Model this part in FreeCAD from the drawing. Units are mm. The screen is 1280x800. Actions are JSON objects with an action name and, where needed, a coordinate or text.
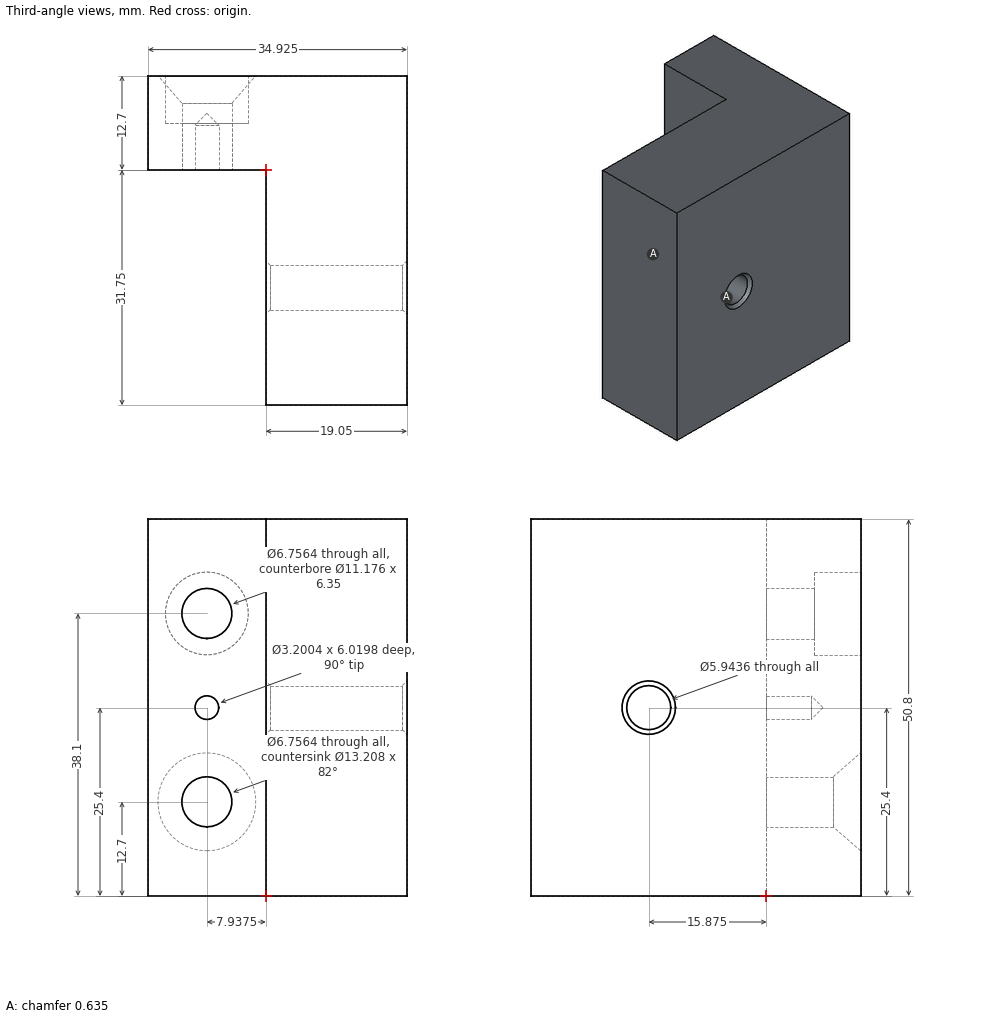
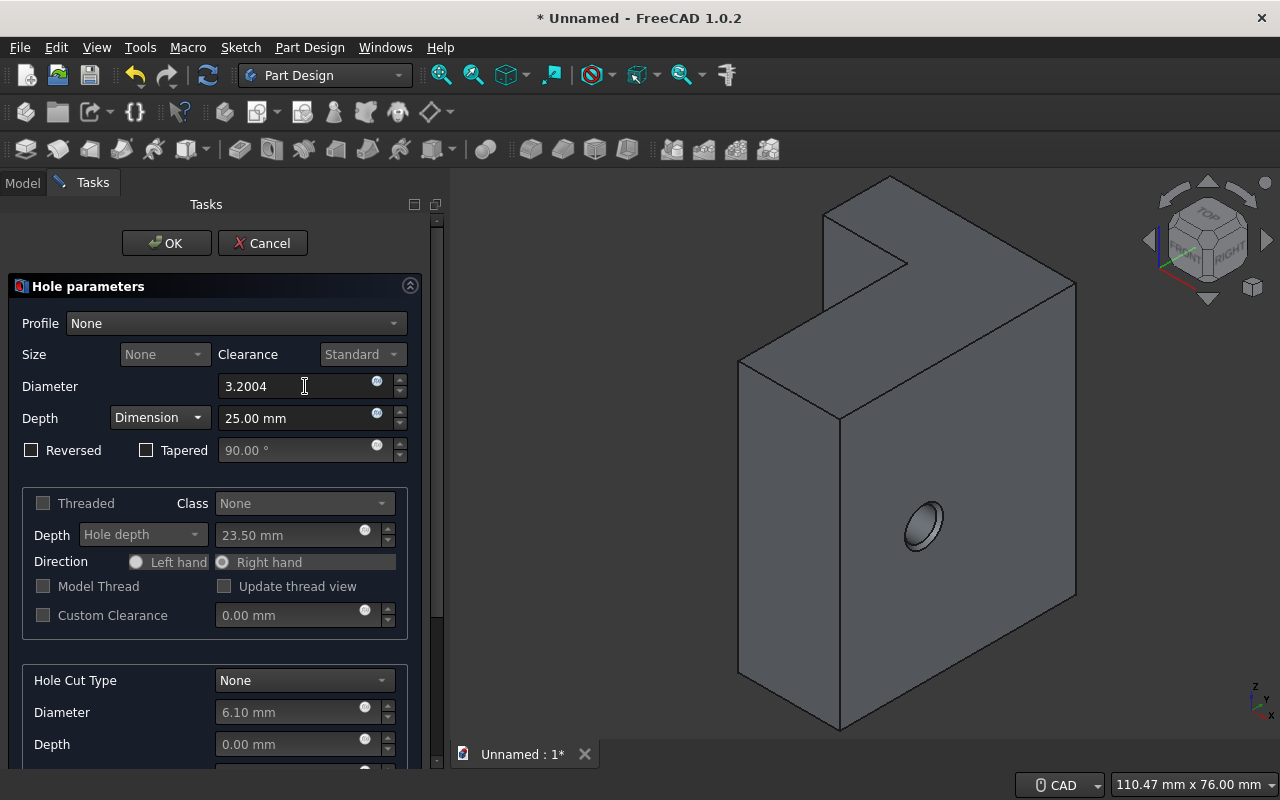
{"action": "triple_click", "coordinate": [305, 418]}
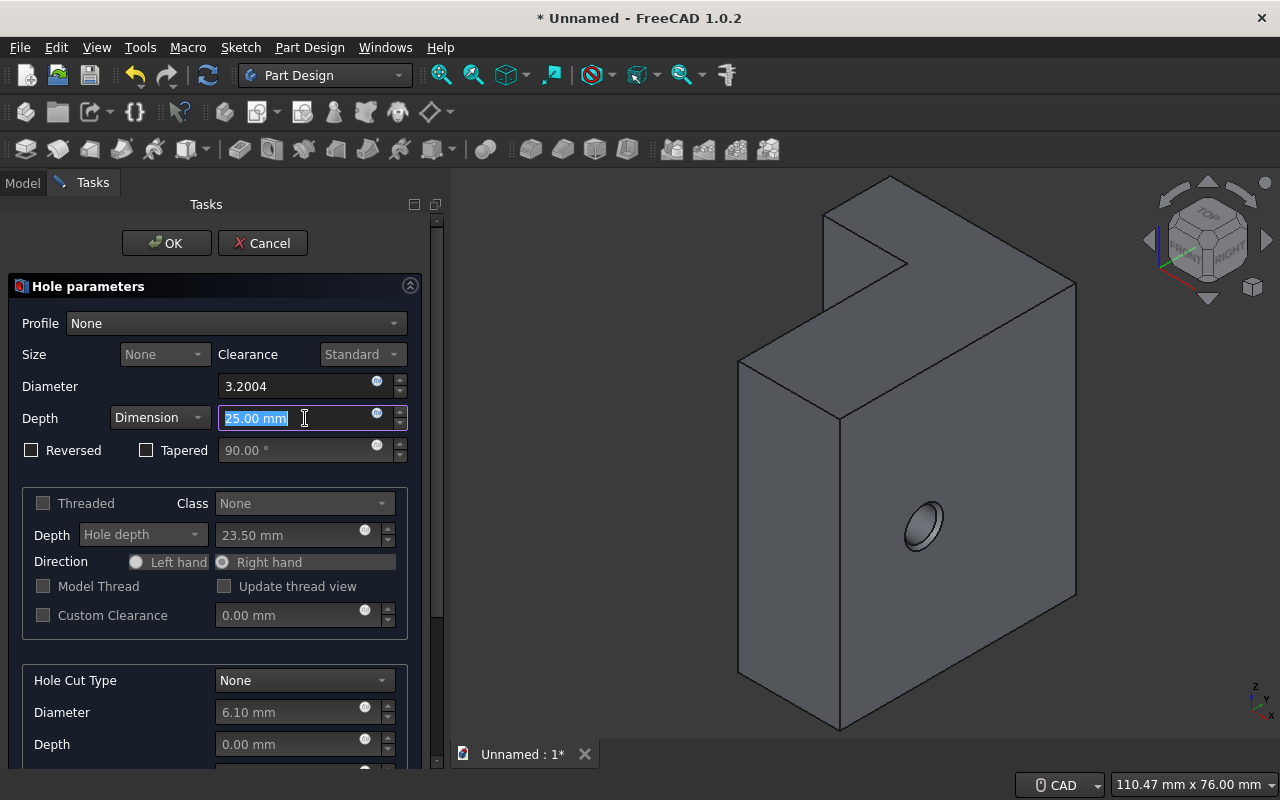
{"action": "type", "text": "6.0198"}
{"action": "key", "text": "Tab"}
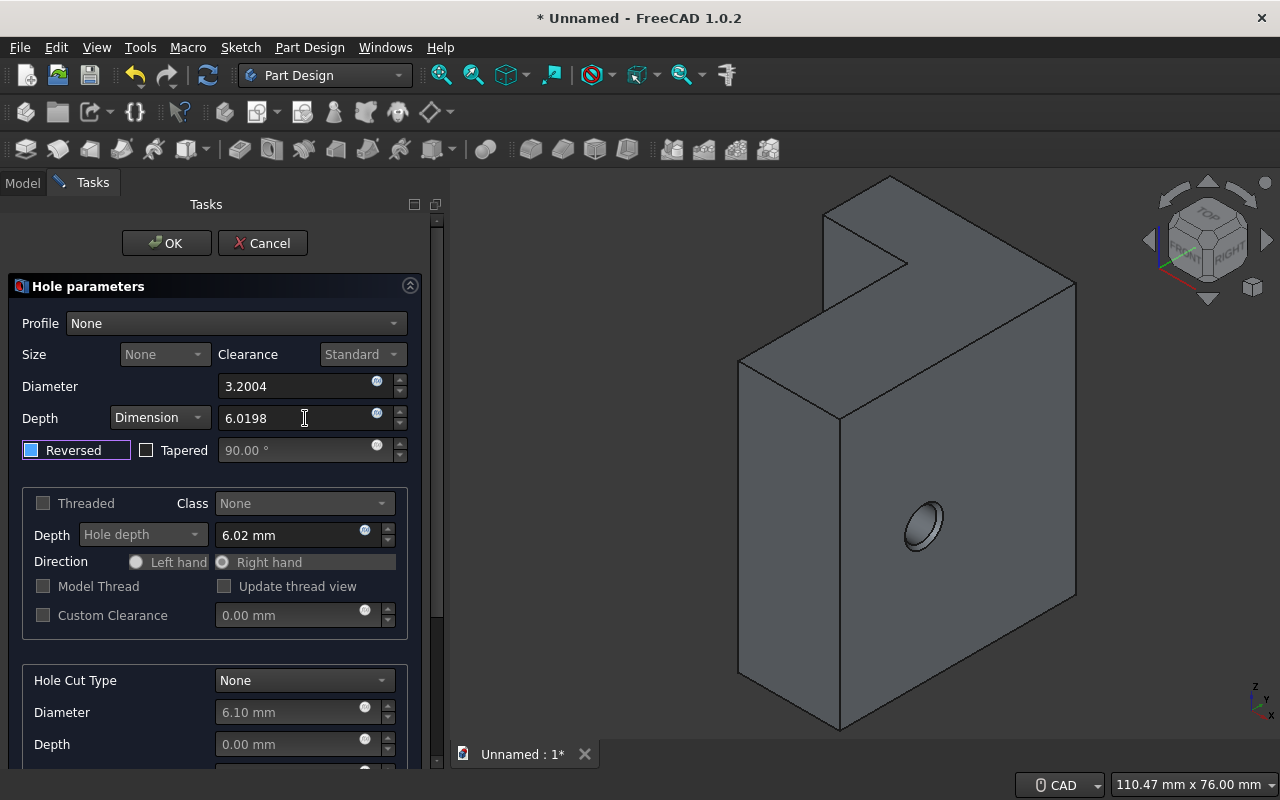
{"action": "scroll", "coordinate": [437, 491], "scroll_direction": "down", "scroll_amount": 4}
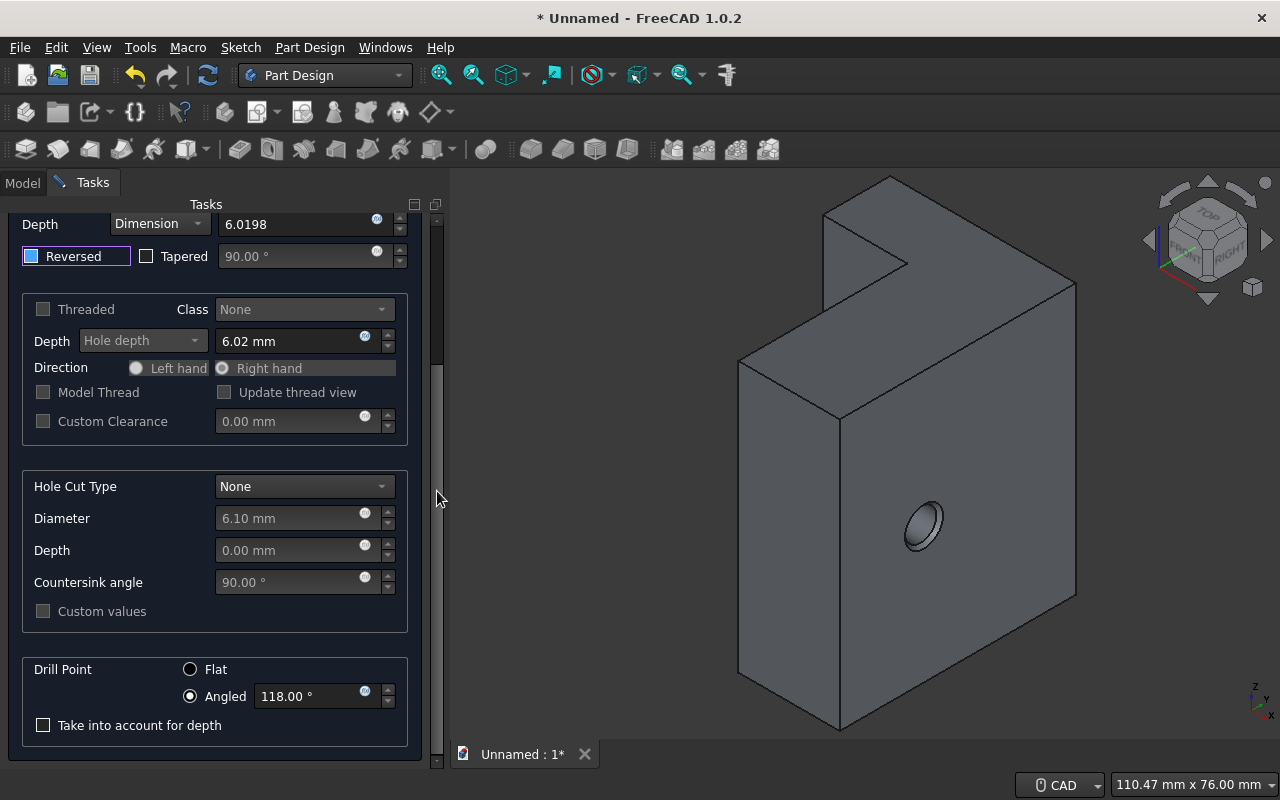
{"action": "triple_click", "coordinate": [317, 696]}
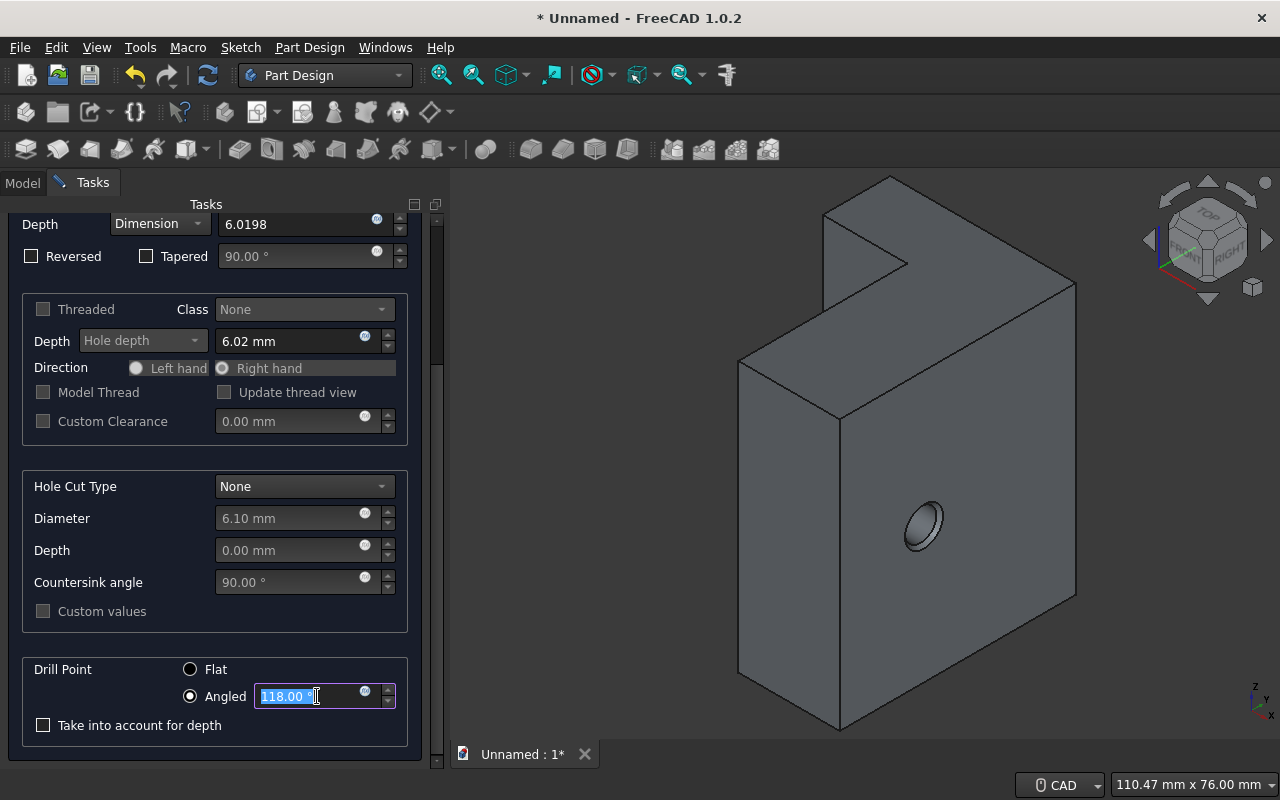
{"action": "type", "text": "90"}
{"action": "key", "text": "Tab"}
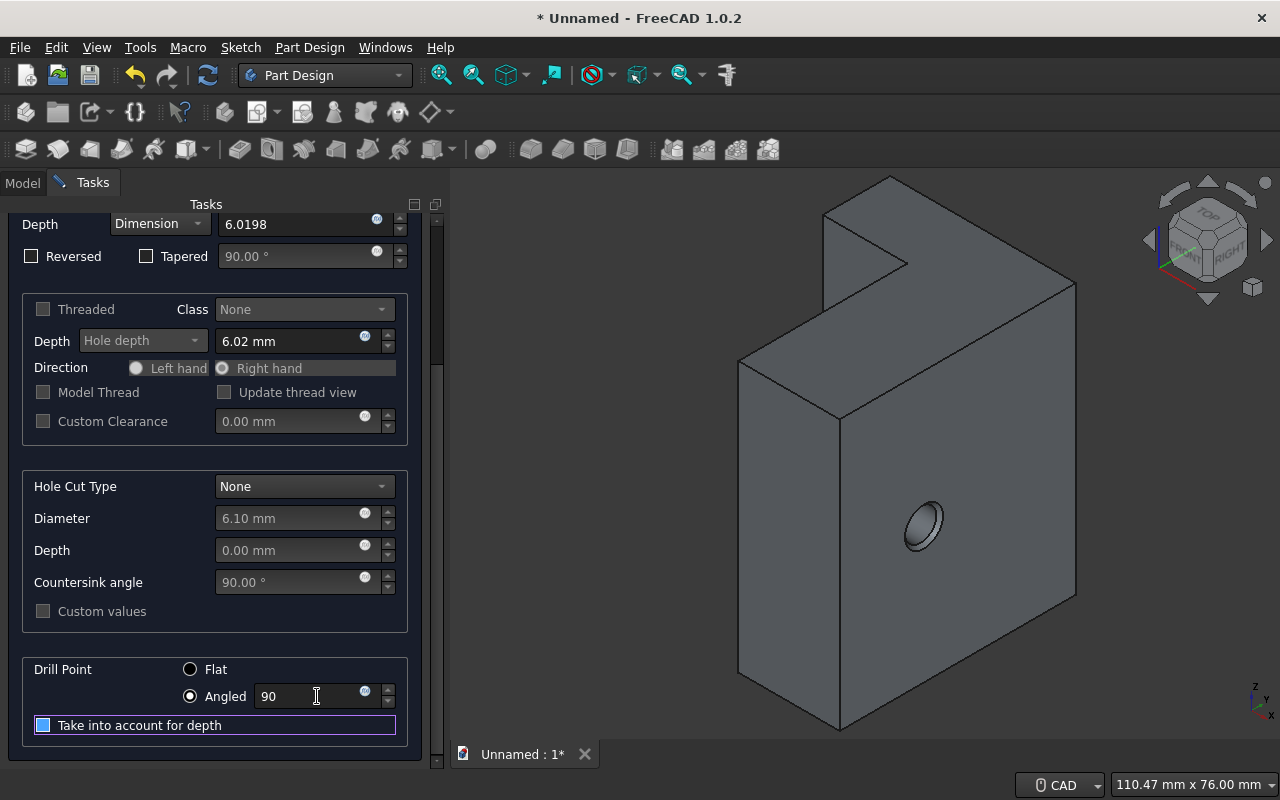
{"action": "scroll", "coordinate": [437, 491], "scroll_direction": "up", "scroll_amount": 4}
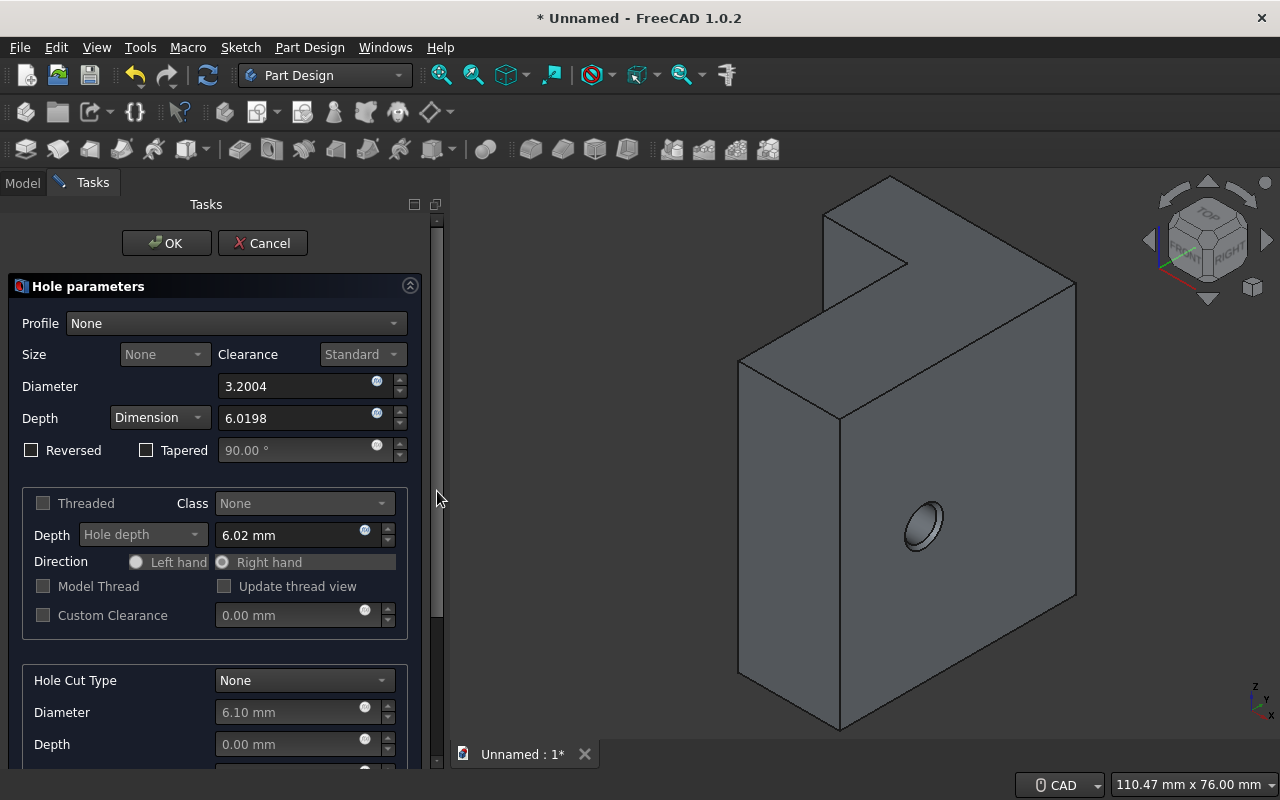
{"action": "left_click", "coordinate": [167, 243]}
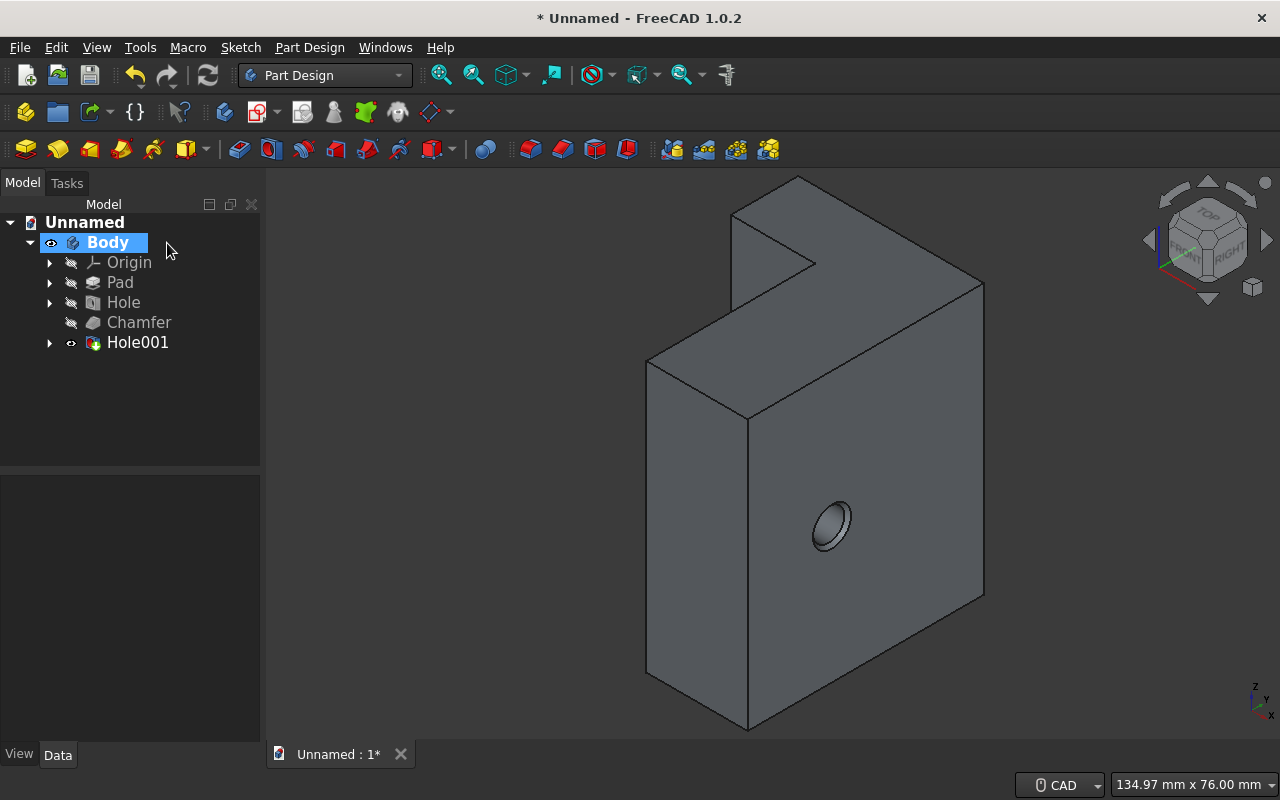
{"action": "key", "text": "4"}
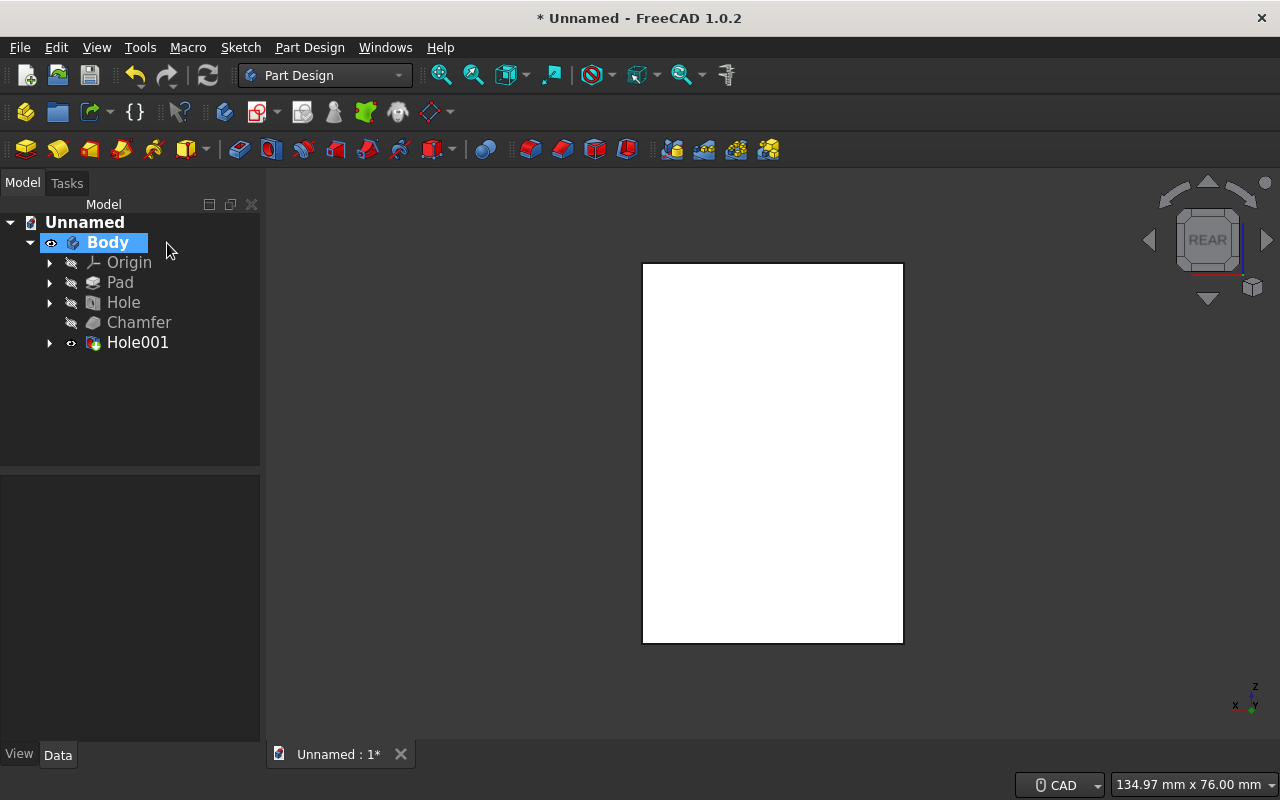
{"action": "left_click", "coordinate": [773, 398]}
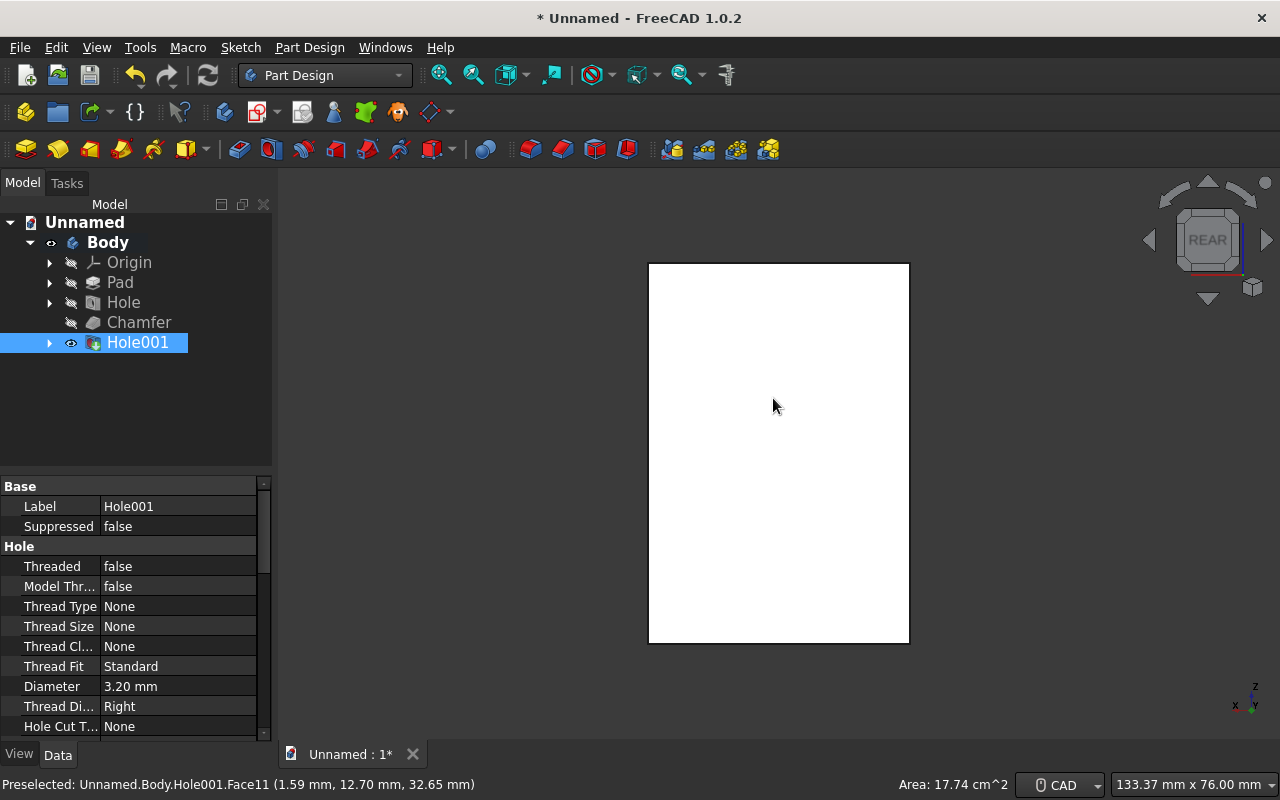
{"action": "left_click", "coordinate": [258, 112]}